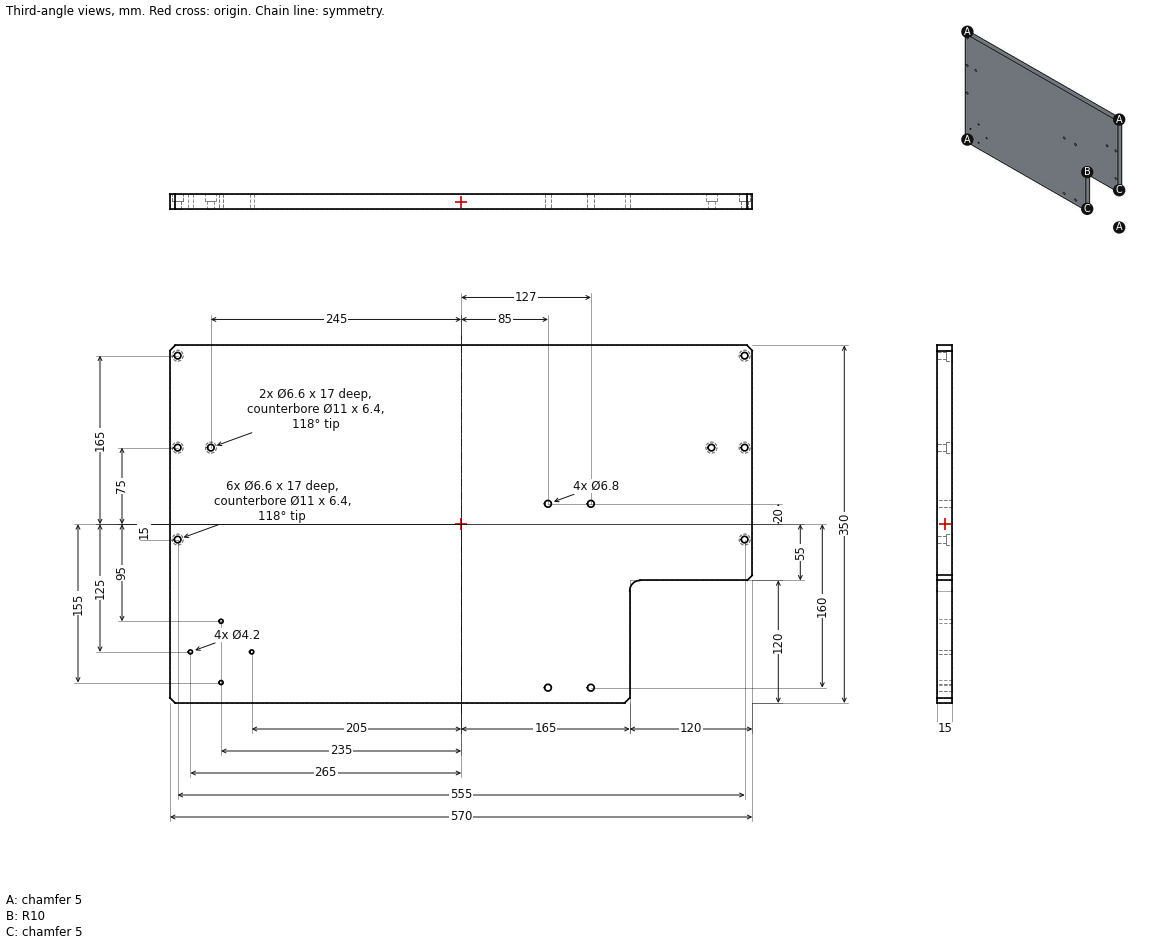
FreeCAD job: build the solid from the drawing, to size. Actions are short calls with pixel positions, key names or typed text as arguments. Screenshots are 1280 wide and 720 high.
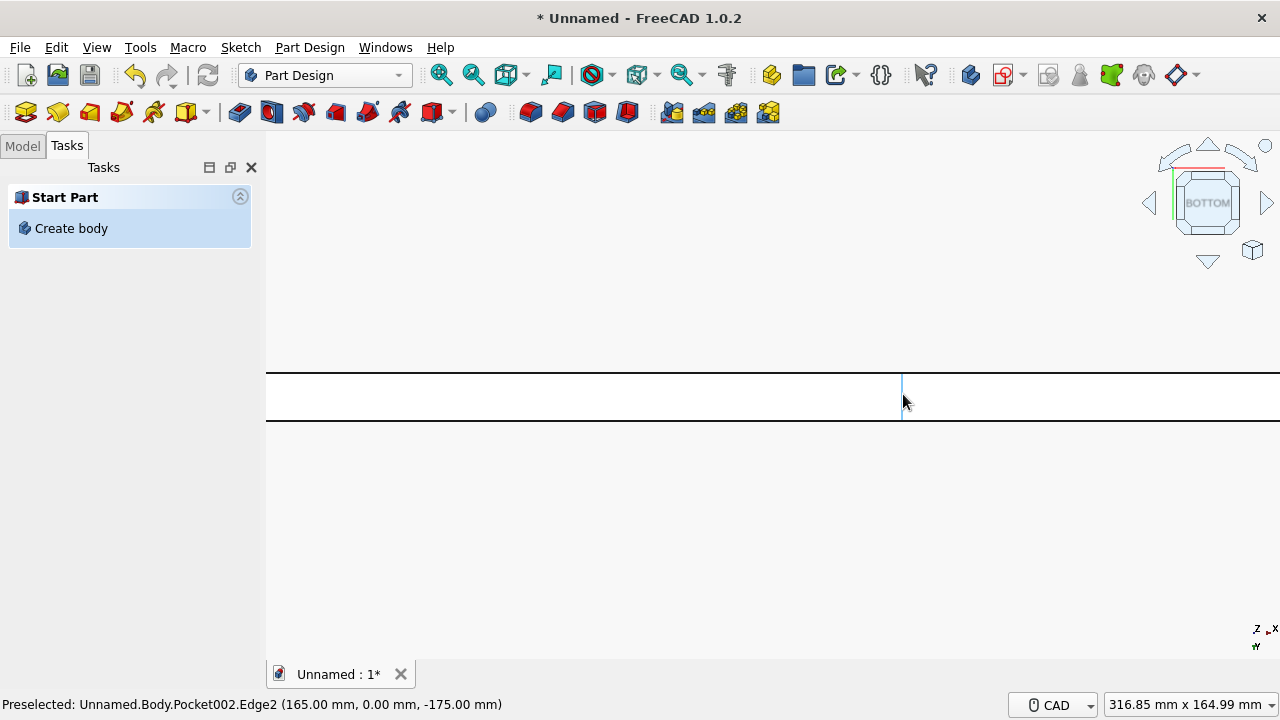
click(442, 76)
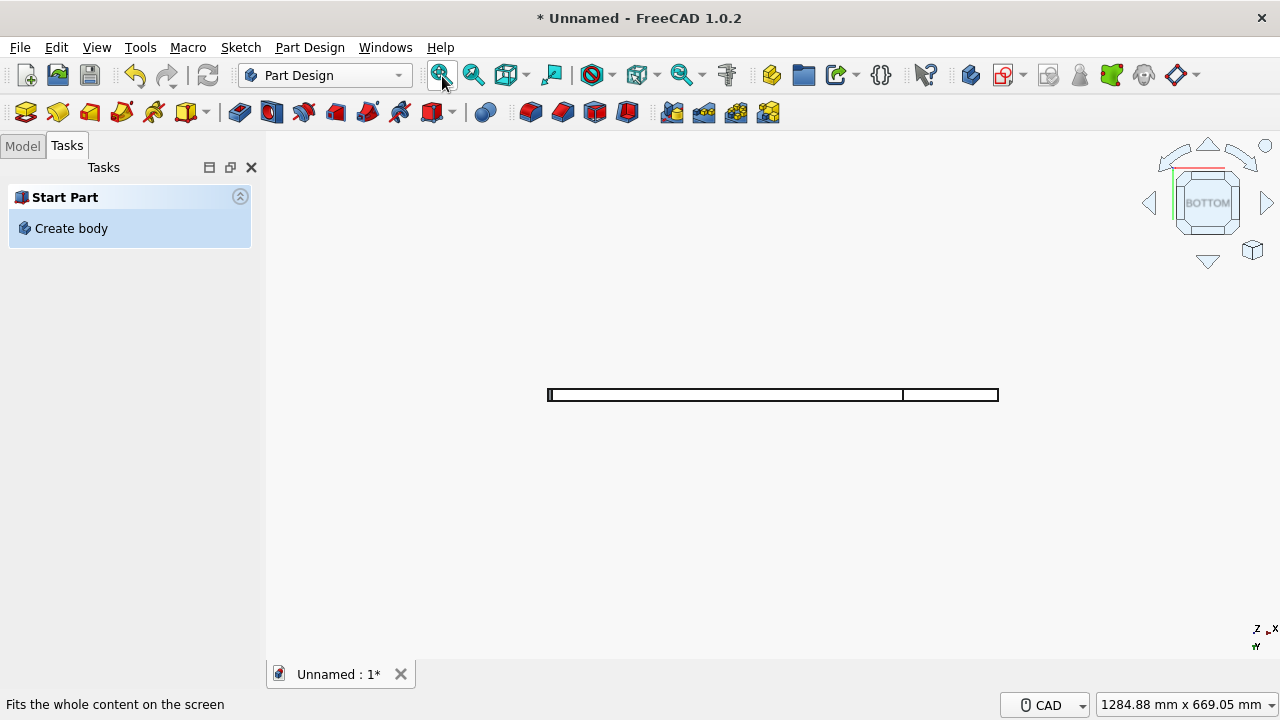
key(4)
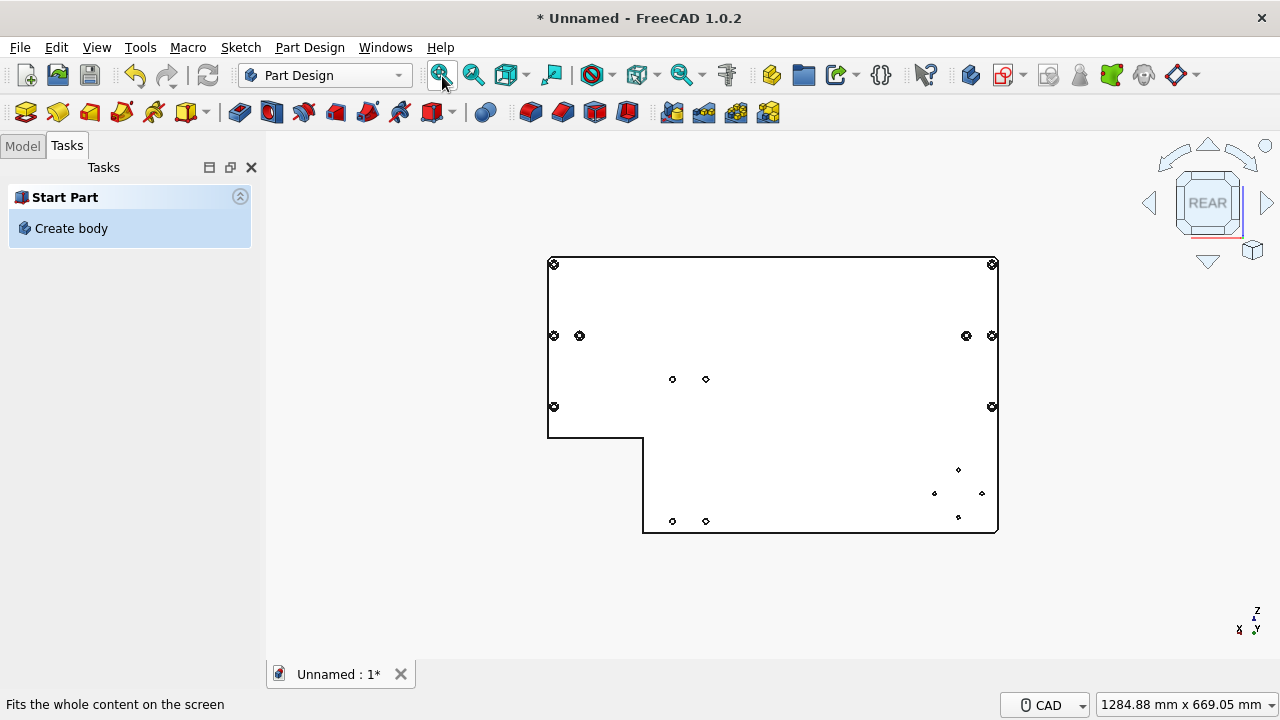
scroll(643, 437, up, 7)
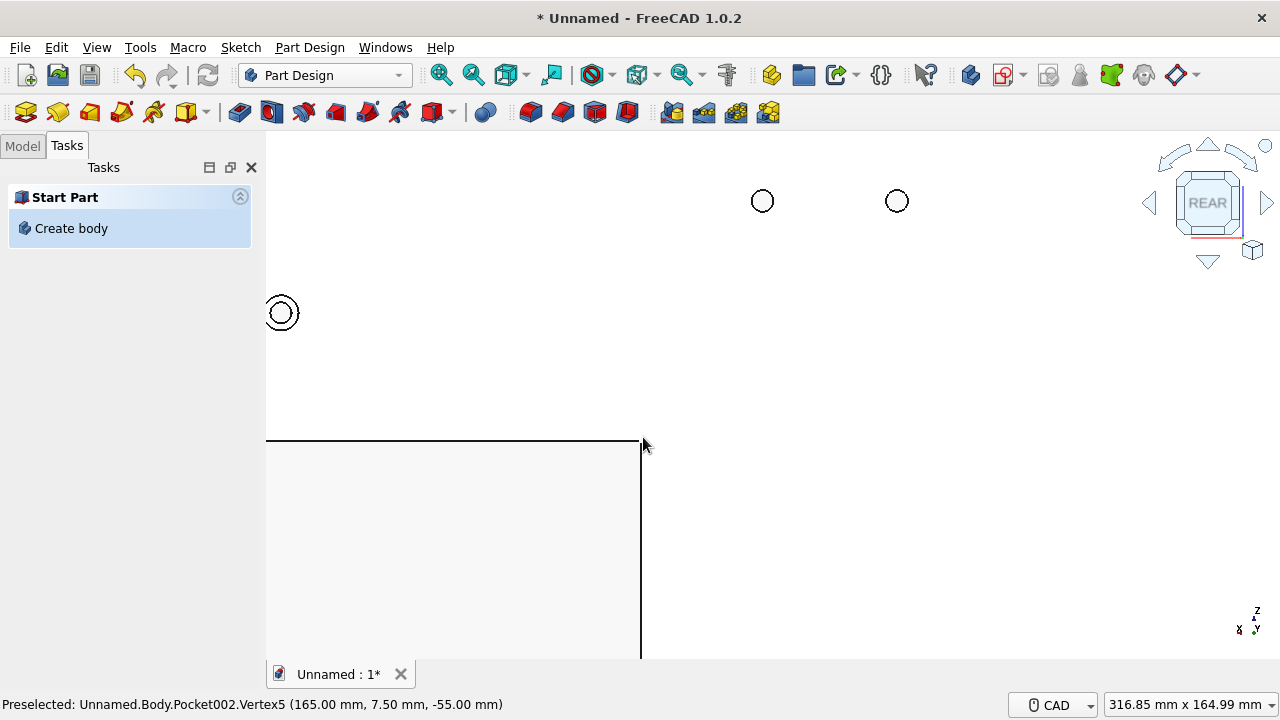
click(442, 76)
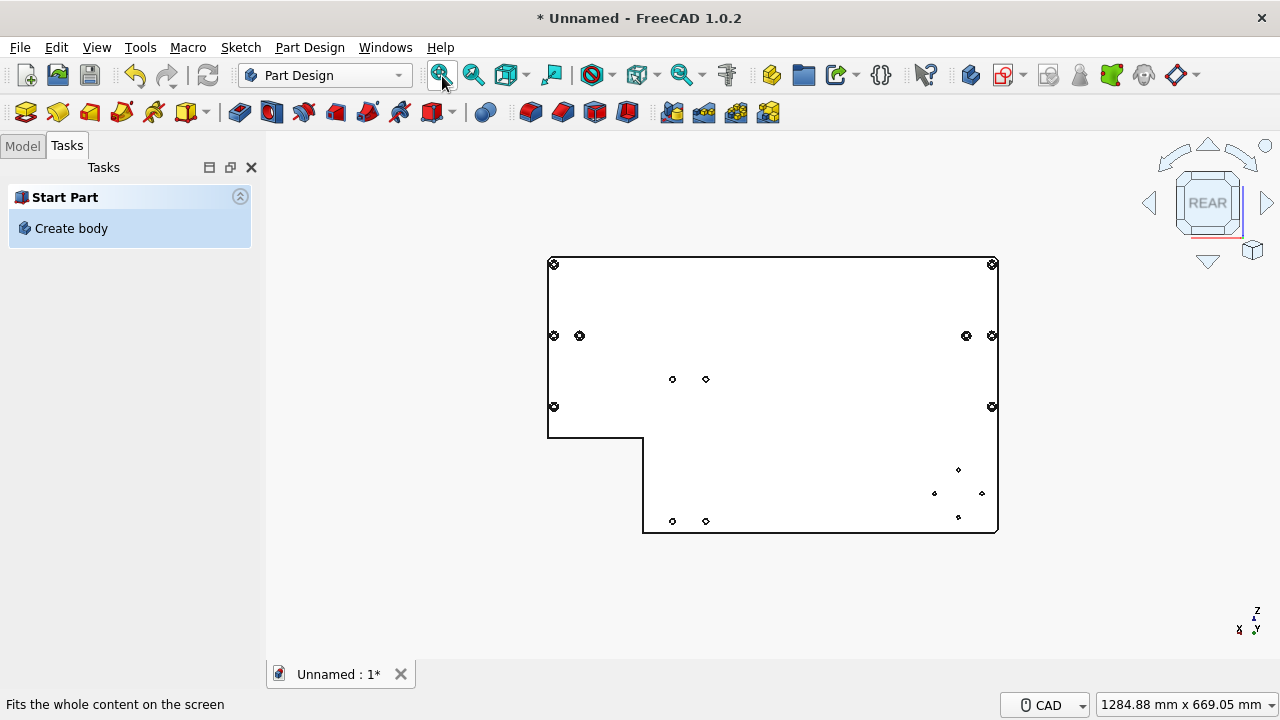
key(6)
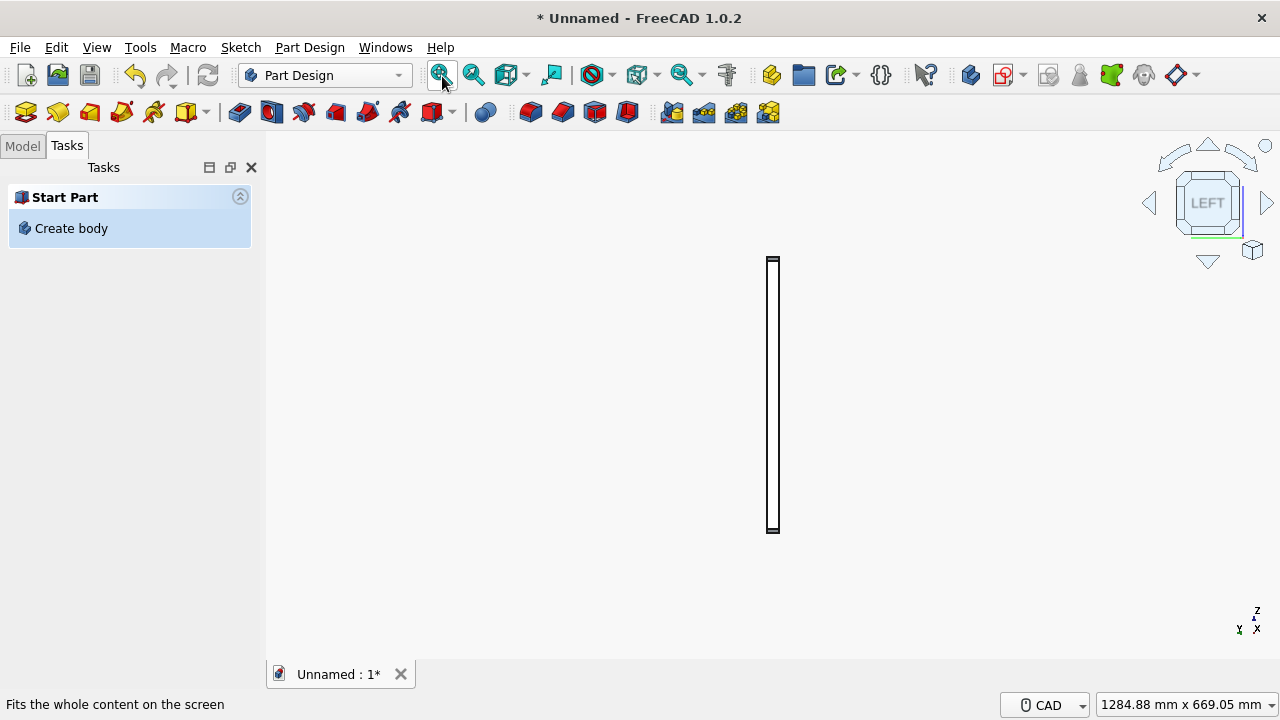
scroll(773, 437, up, 7)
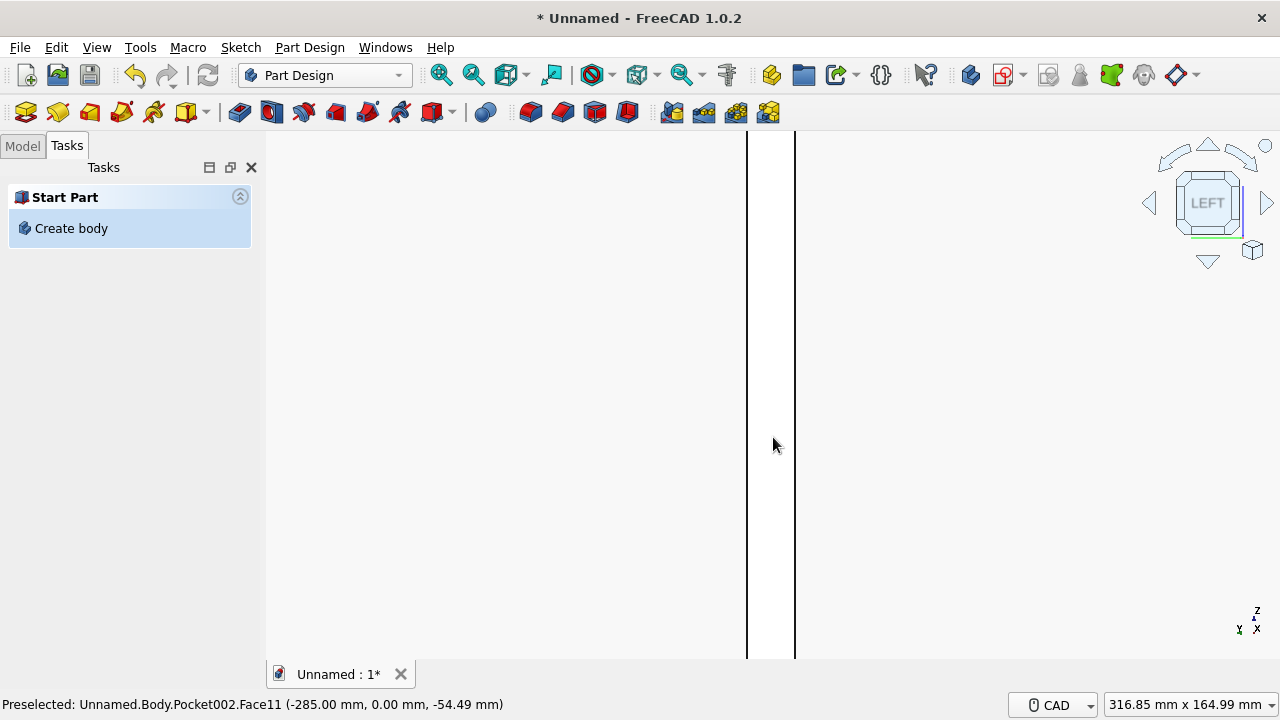
click(442, 76)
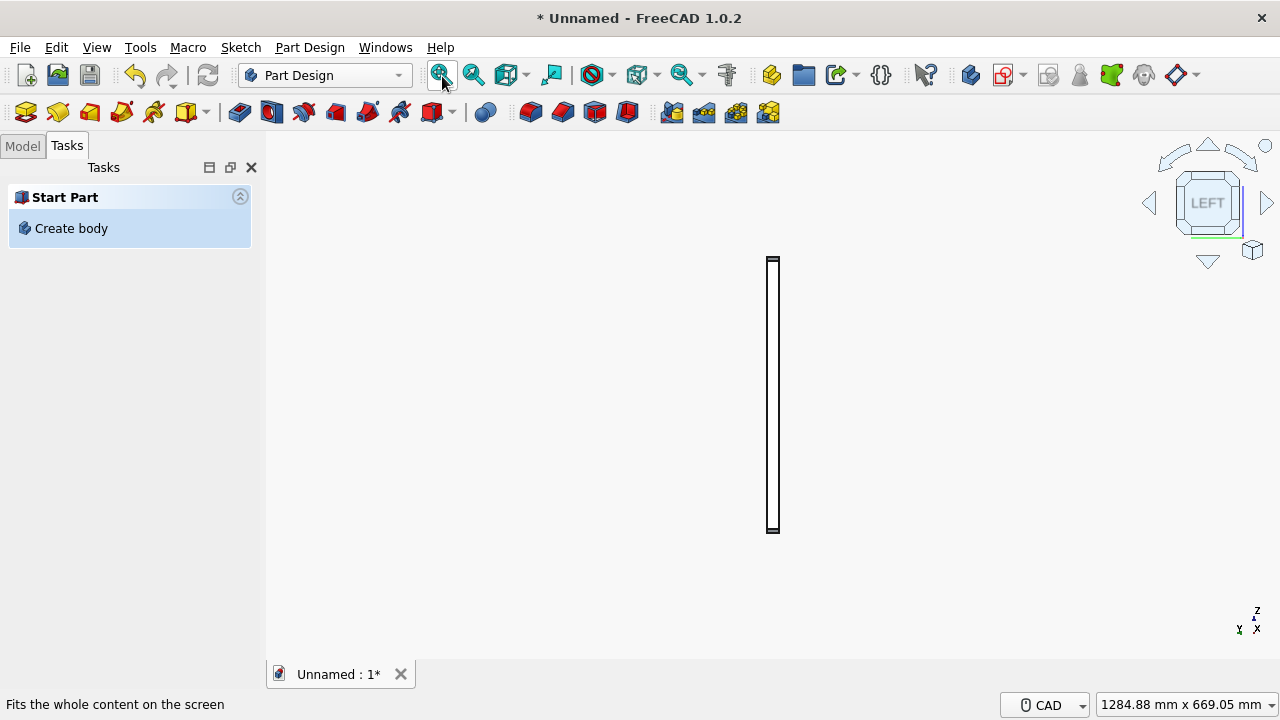
key(v)
key(3)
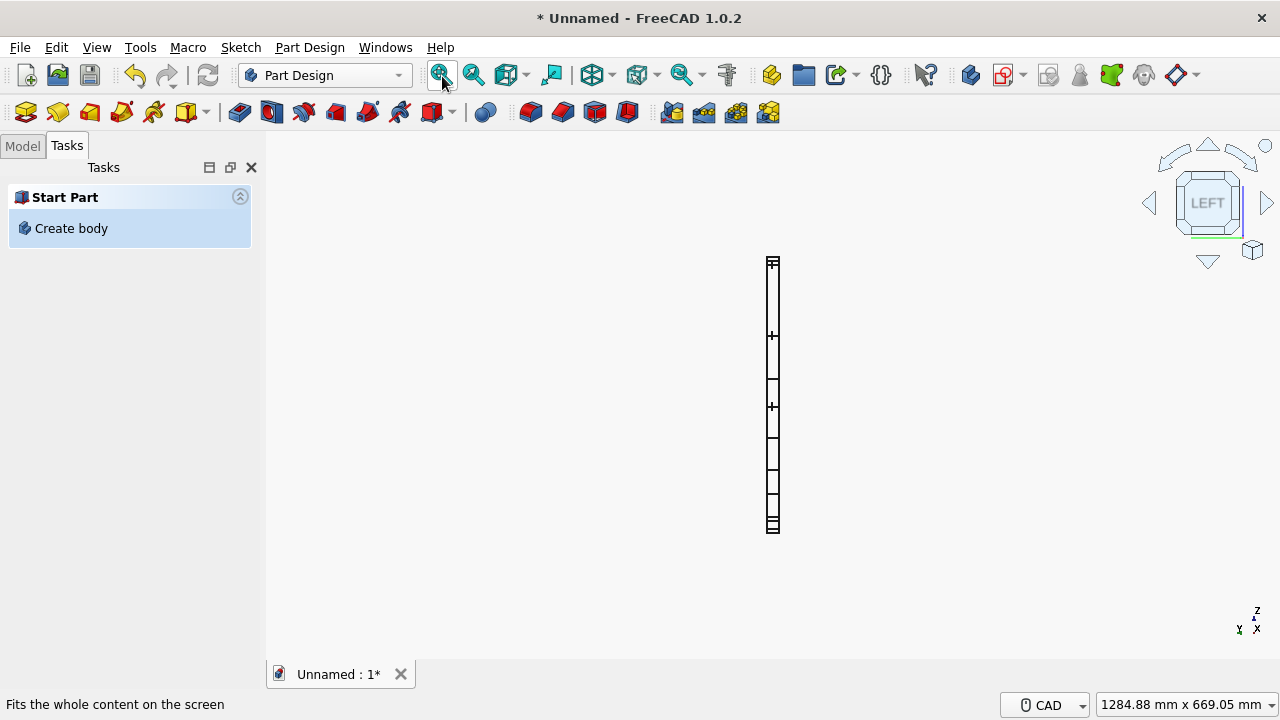
key(0)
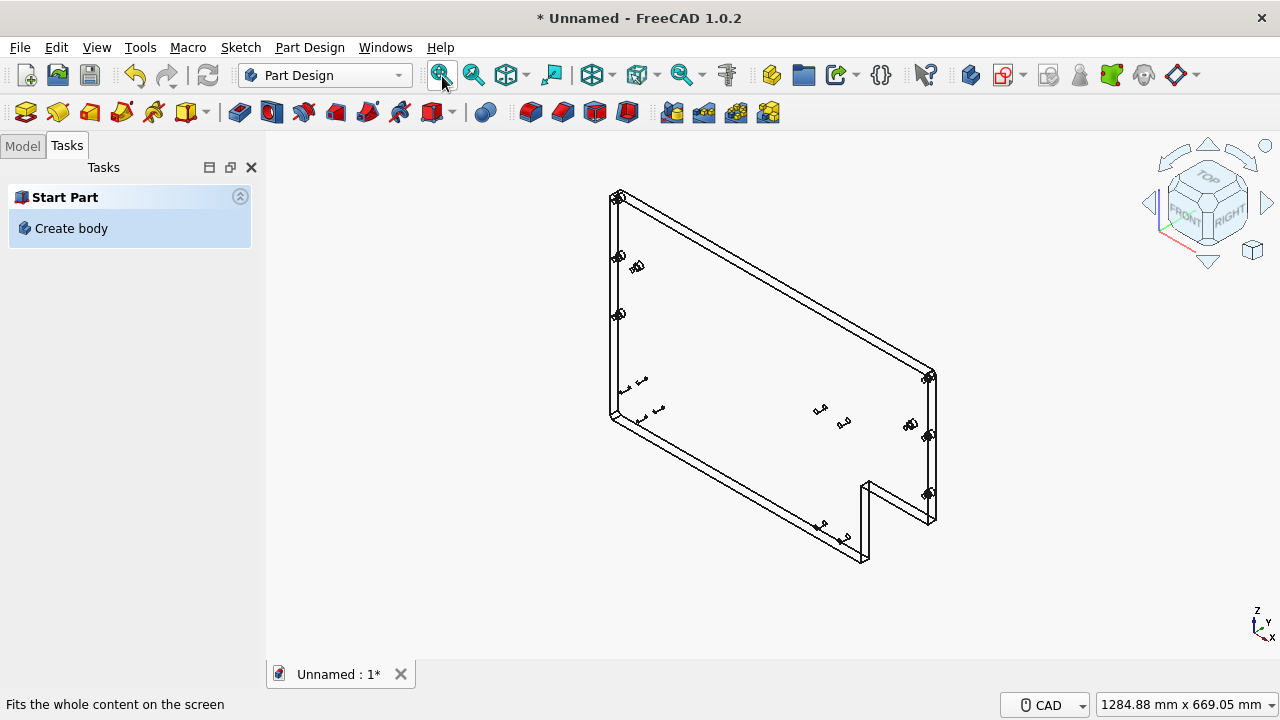
click(868, 481)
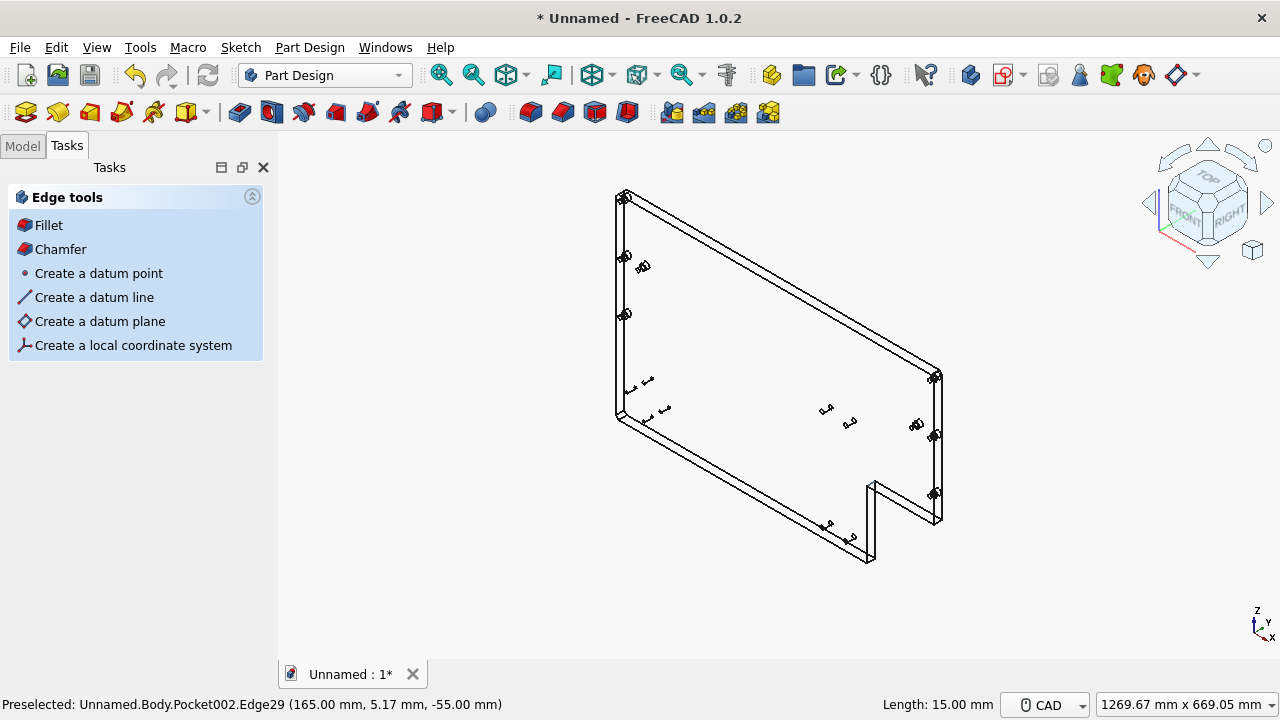
key(v)
key(1)